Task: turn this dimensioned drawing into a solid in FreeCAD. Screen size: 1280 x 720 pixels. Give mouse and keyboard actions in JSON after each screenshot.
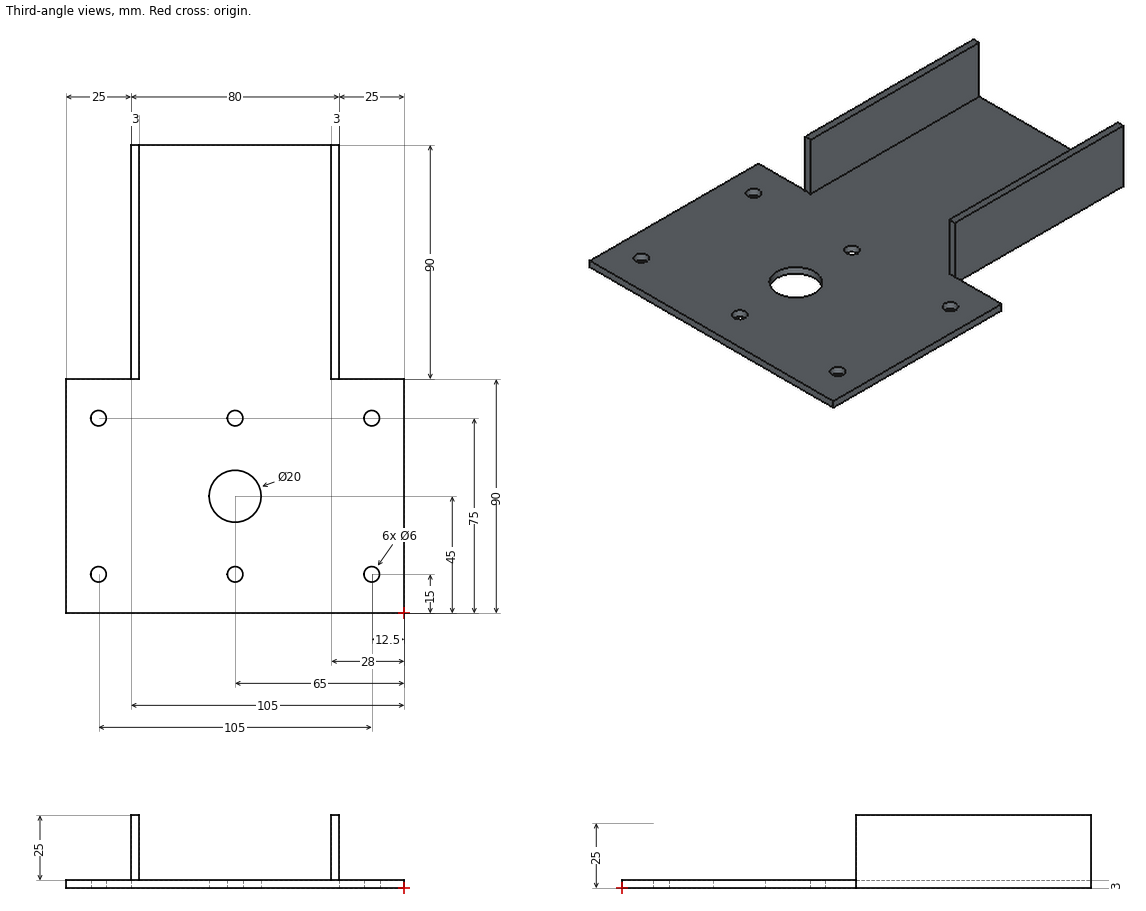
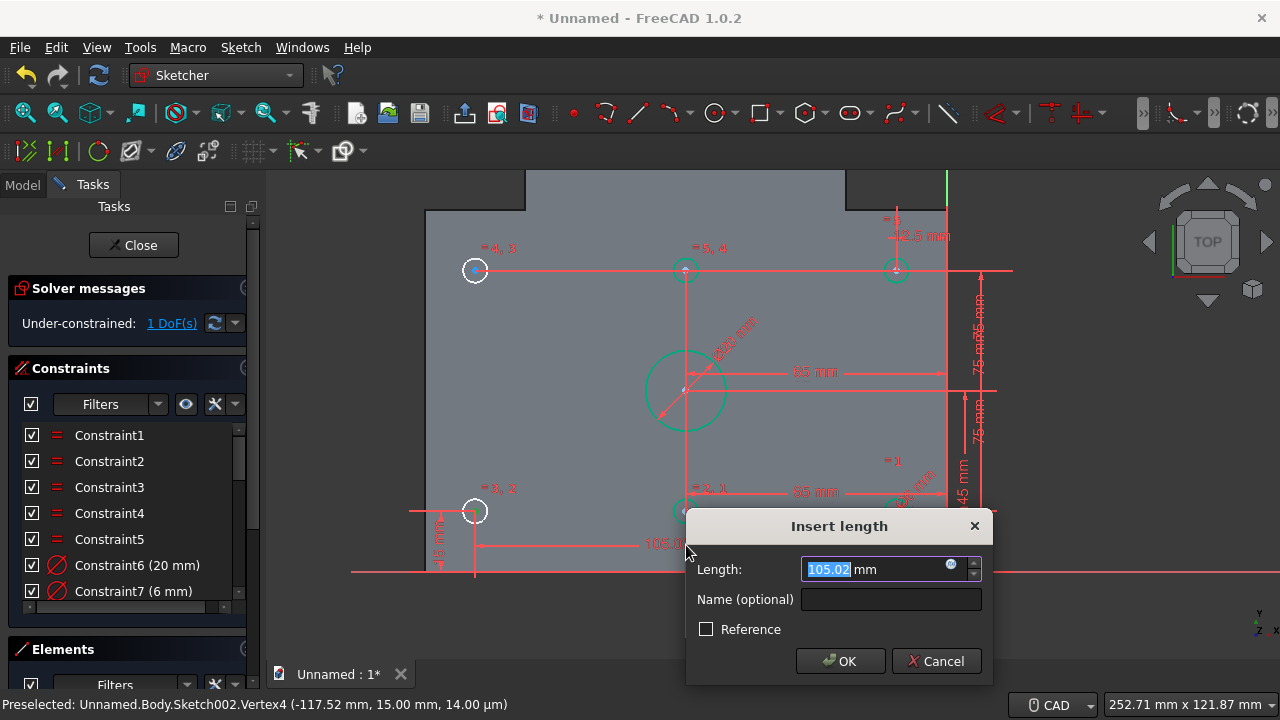
{"action": "type", "text": "105"}
{"action": "key", "text": "Return"}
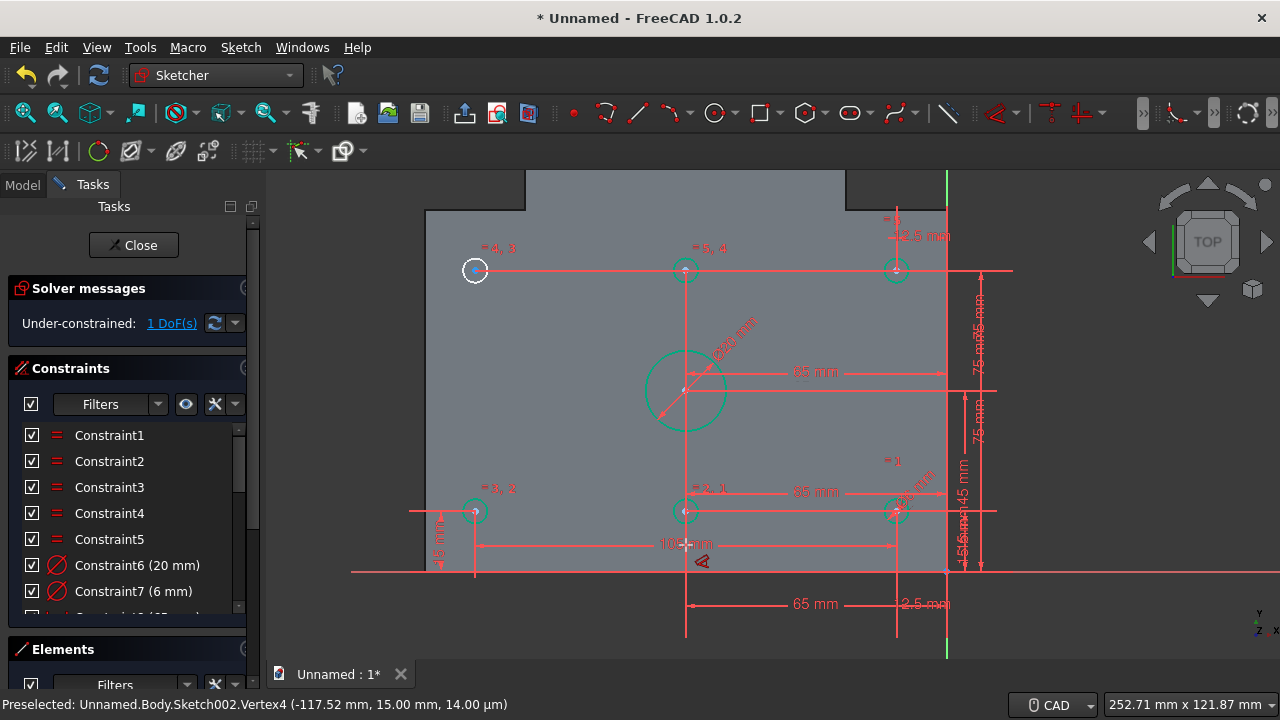
{"action": "left_click", "coordinate": [897, 511]}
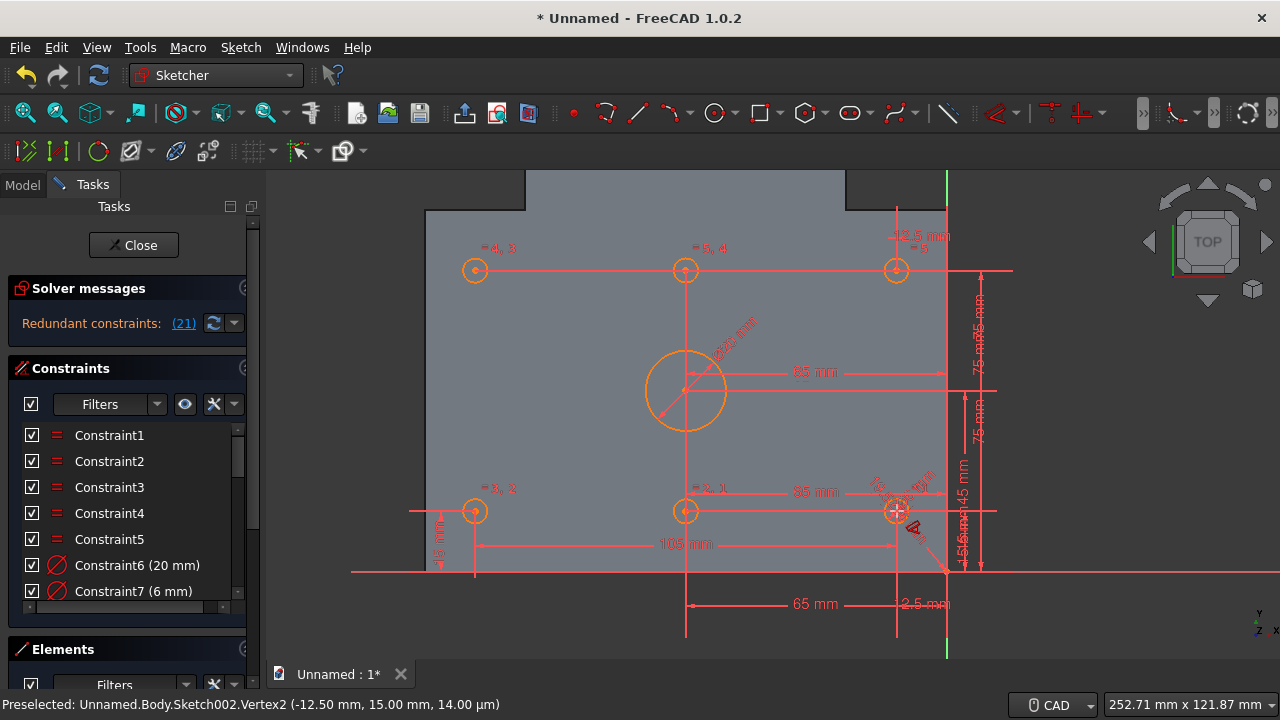
{"action": "left_click", "coordinate": [475, 271]}
{"action": "left_click", "coordinate": [686, 237]}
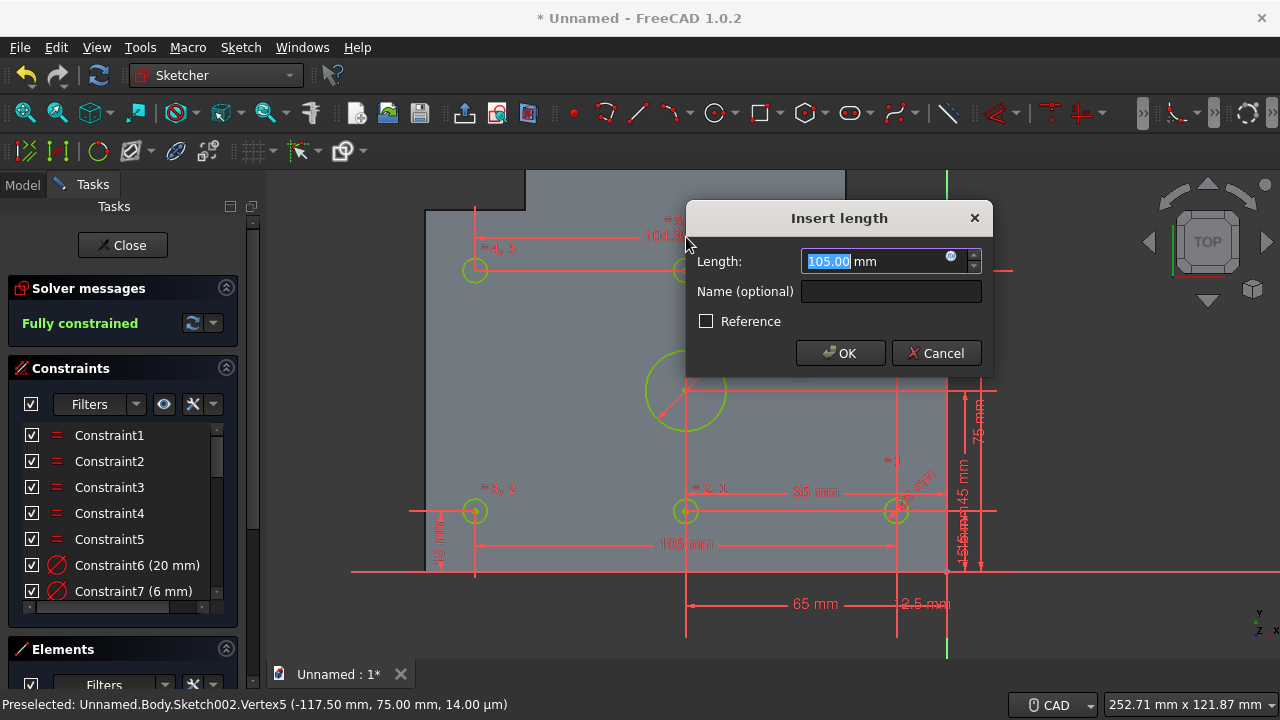
{"action": "type", "text": "105"}
{"action": "key", "text": "Return"}
{"action": "key", "text": "Escape"}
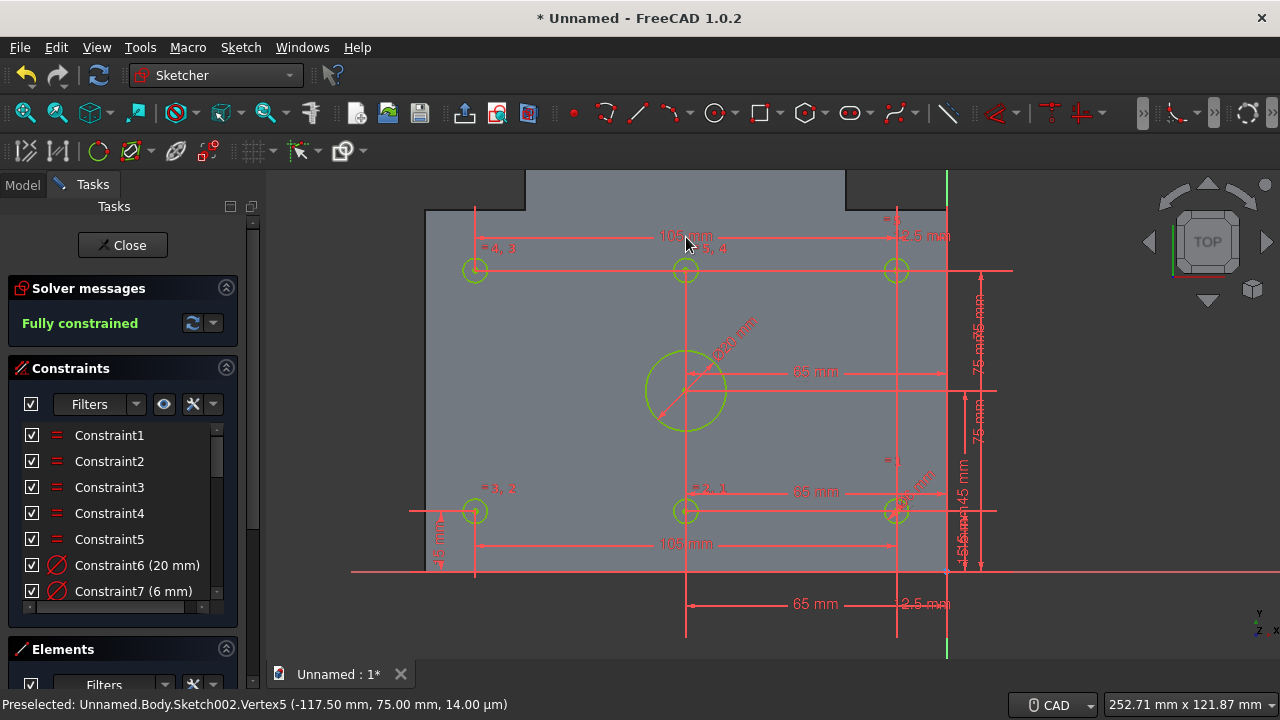
{"action": "left_click", "coordinate": [123, 245]}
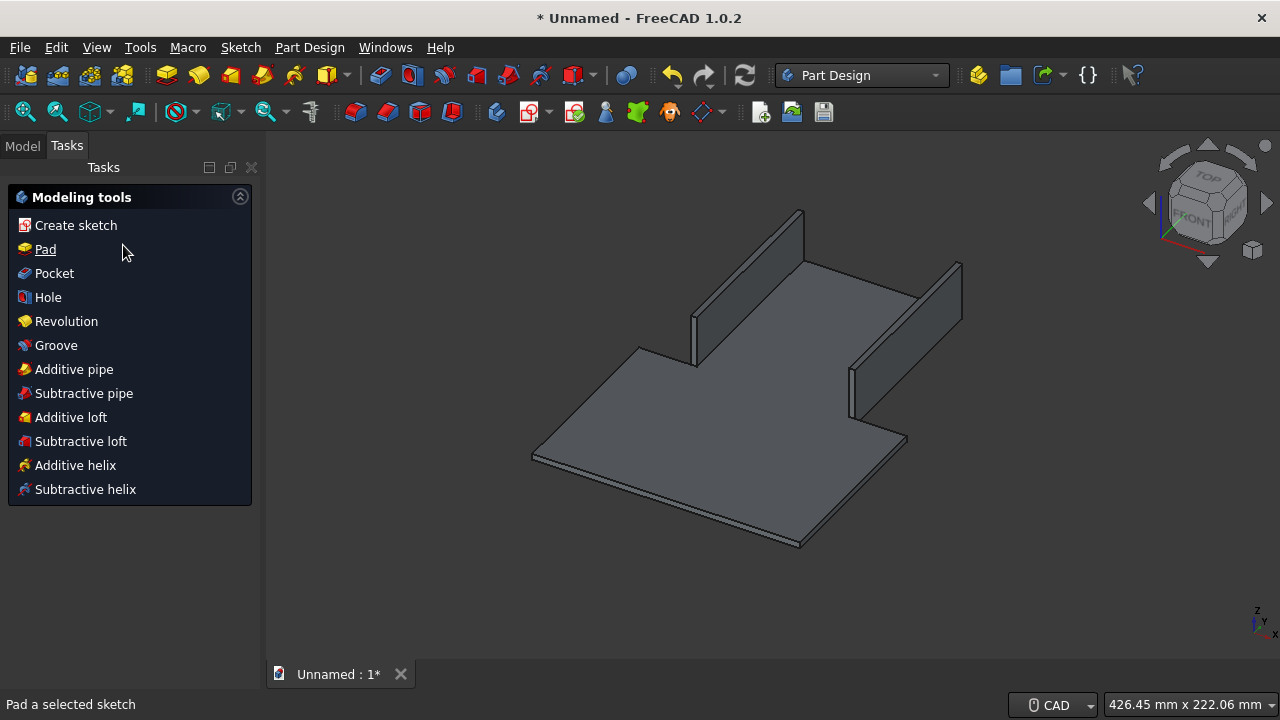
{"action": "left_click", "coordinate": [382, 76]}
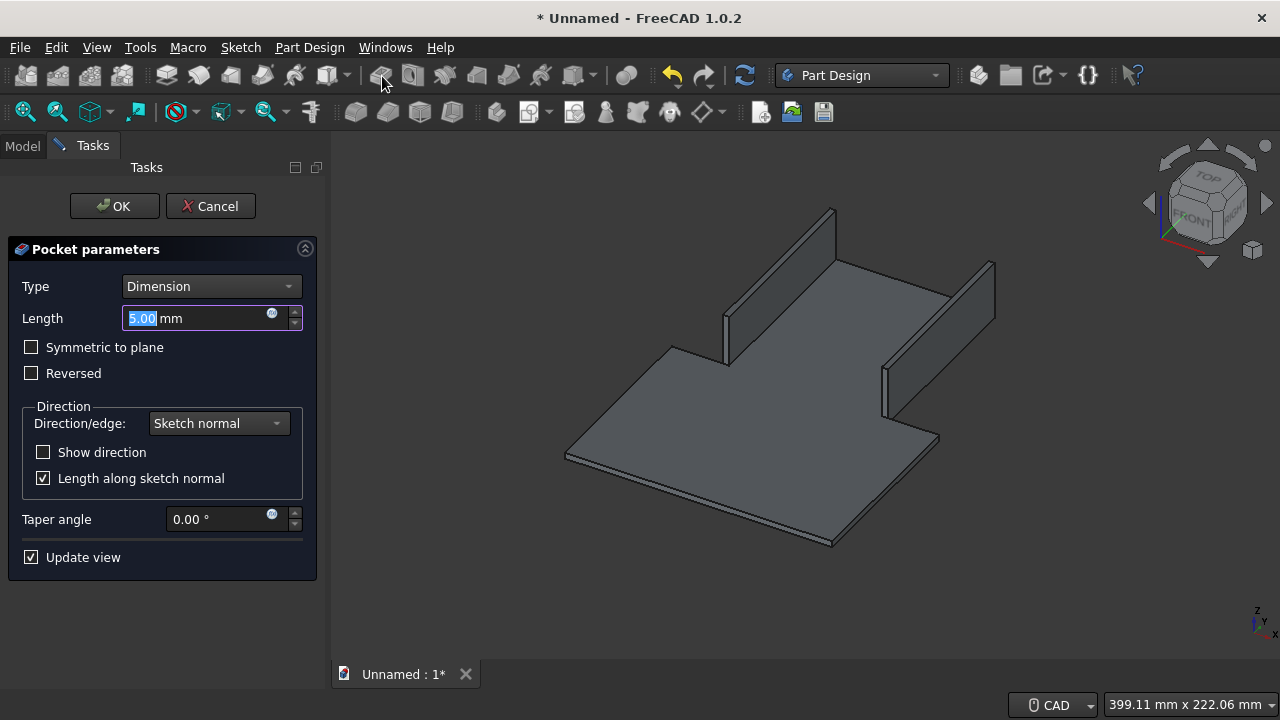
{"action": "type", "text": "25"}
{"action": "key", "text": "Tab"}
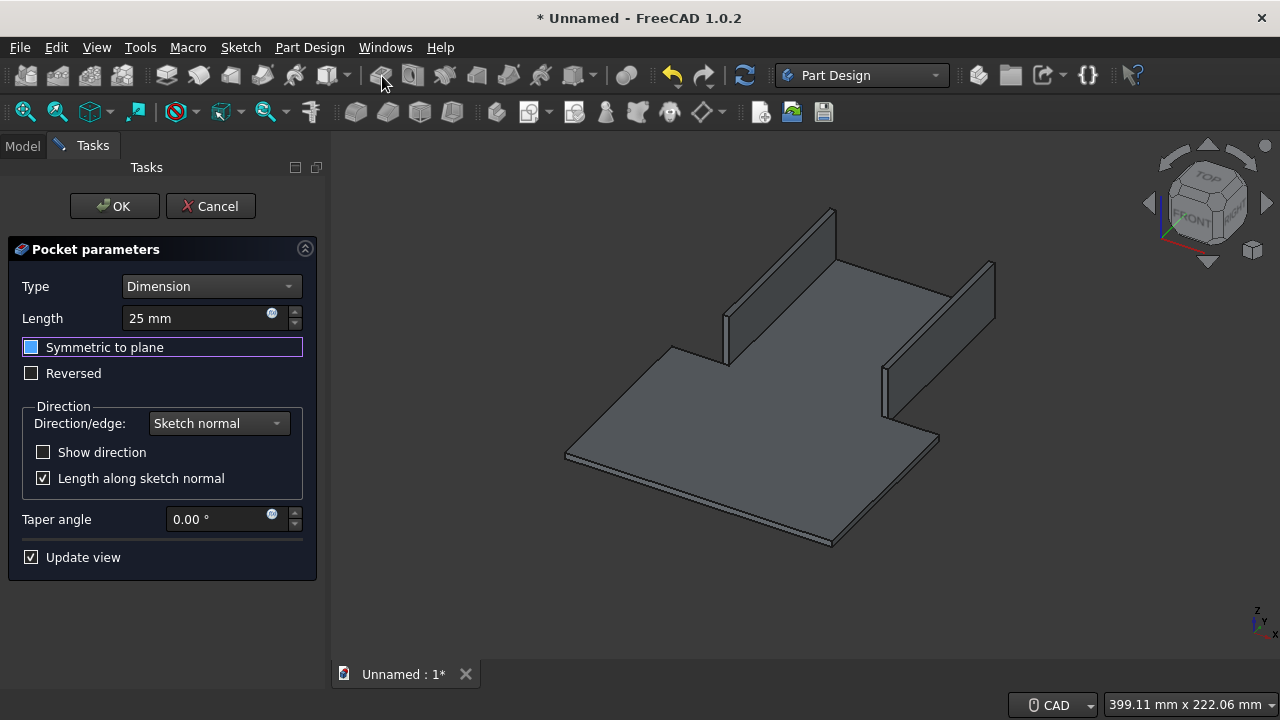
{"action": "left_click", "coordinate": [30, 373]}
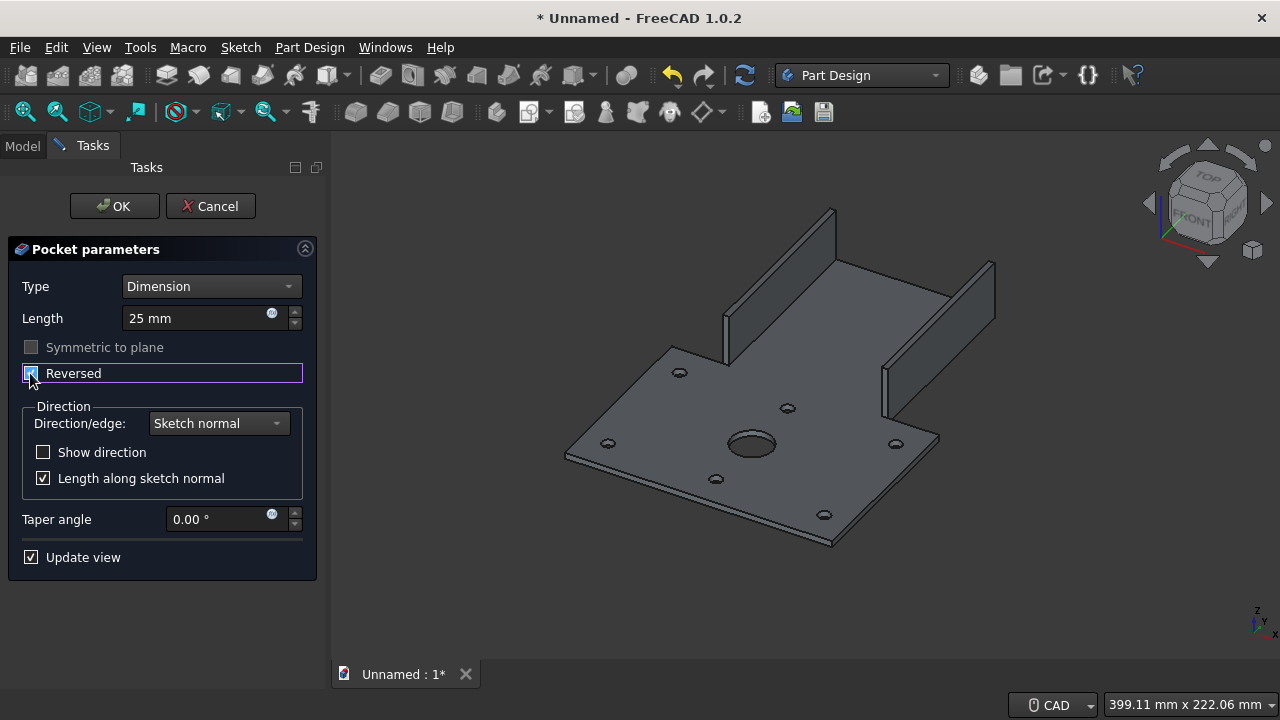
{"action": "left_click", "coordinate": [115, 206]}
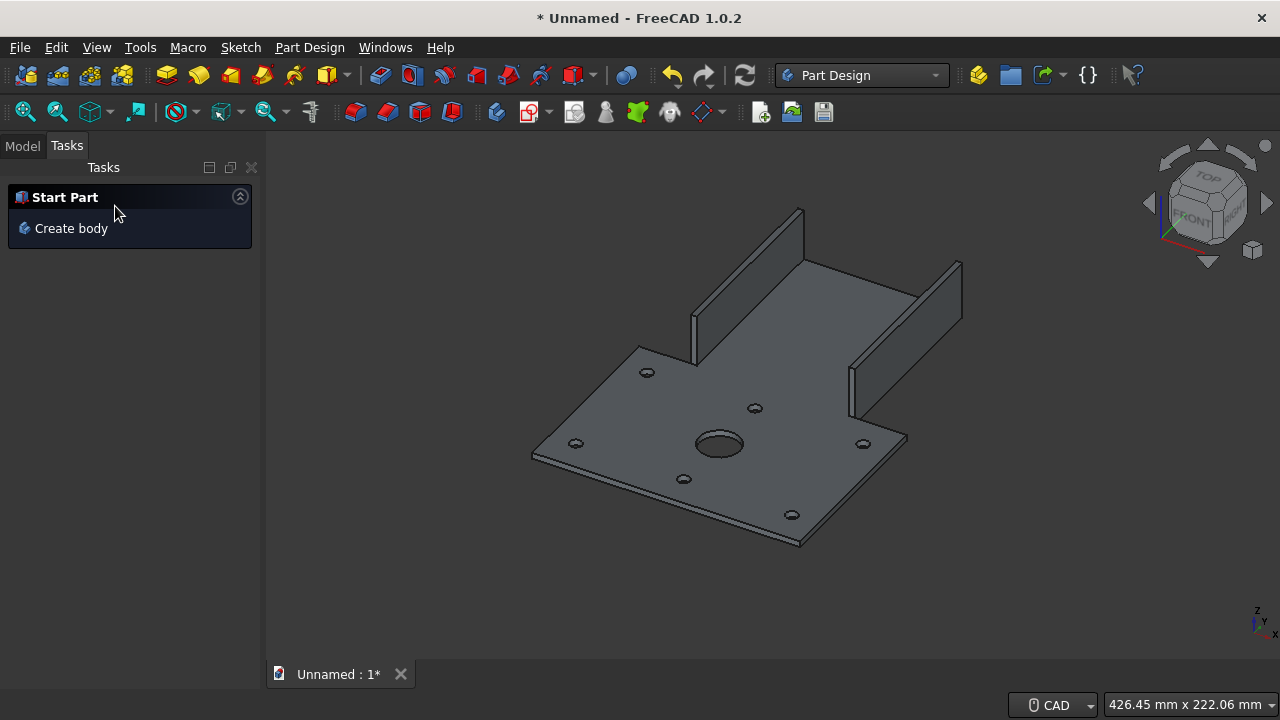
{"action": "key", "text": "0"}